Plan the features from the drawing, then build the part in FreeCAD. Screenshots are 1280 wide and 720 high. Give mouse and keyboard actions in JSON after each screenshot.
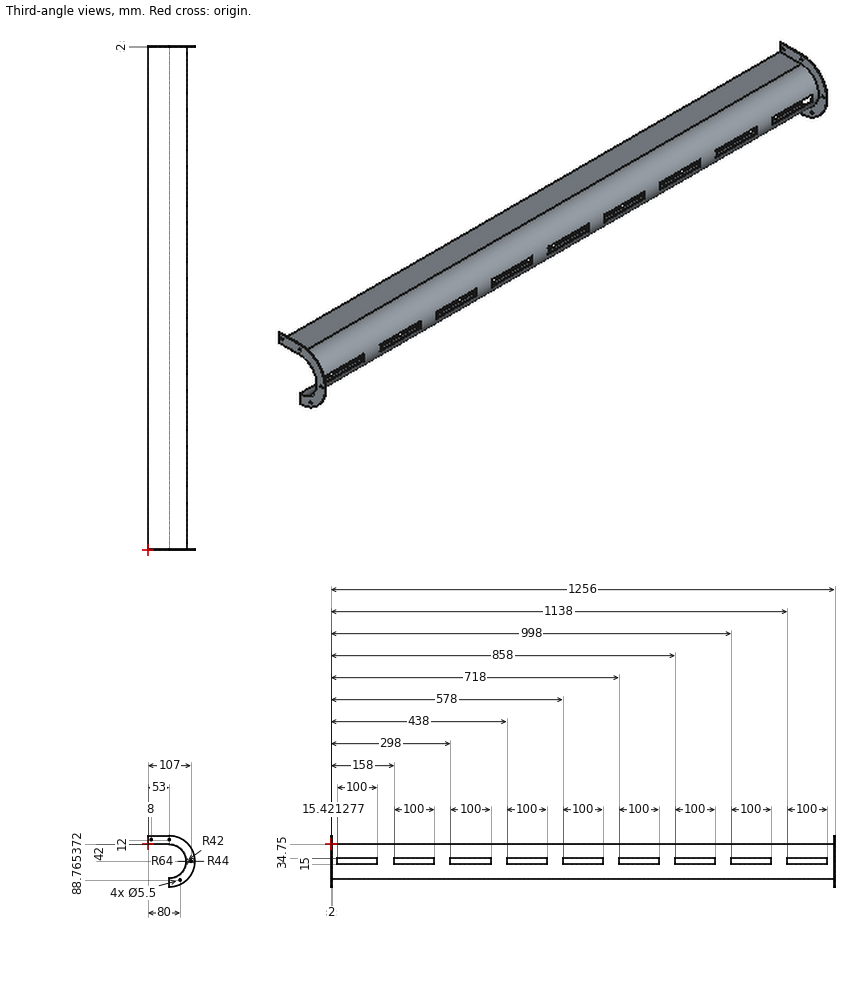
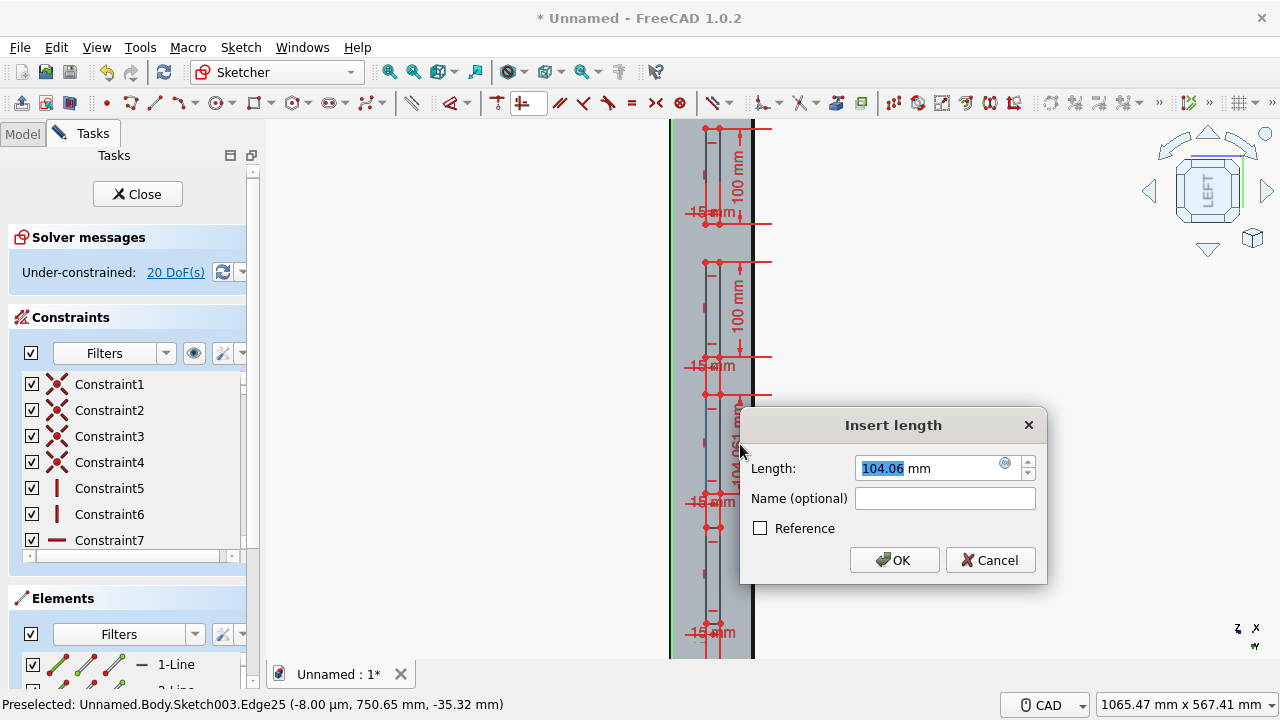
{"action": "type", "text": "100"}
{"action": "key", "text": "Return"}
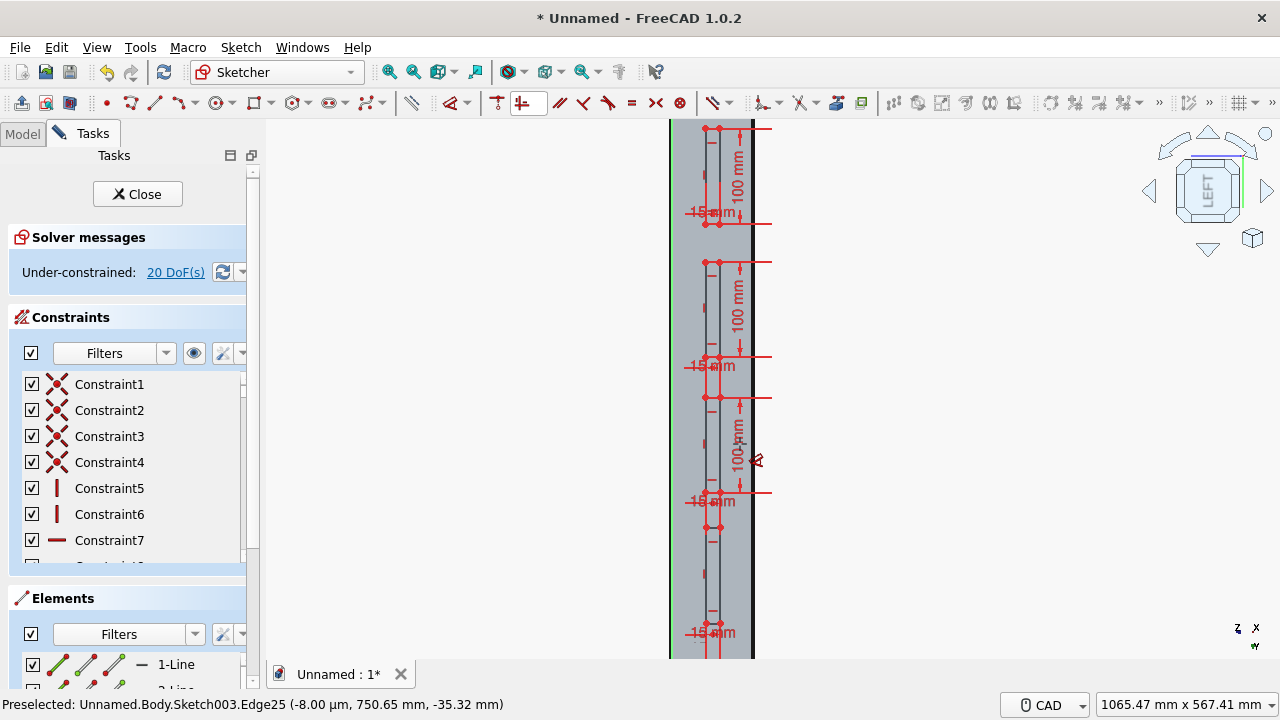
{"action": "left_click", "coordinate": [706, 557]}
{"action": "left_click", "coordinate": [740, 576]}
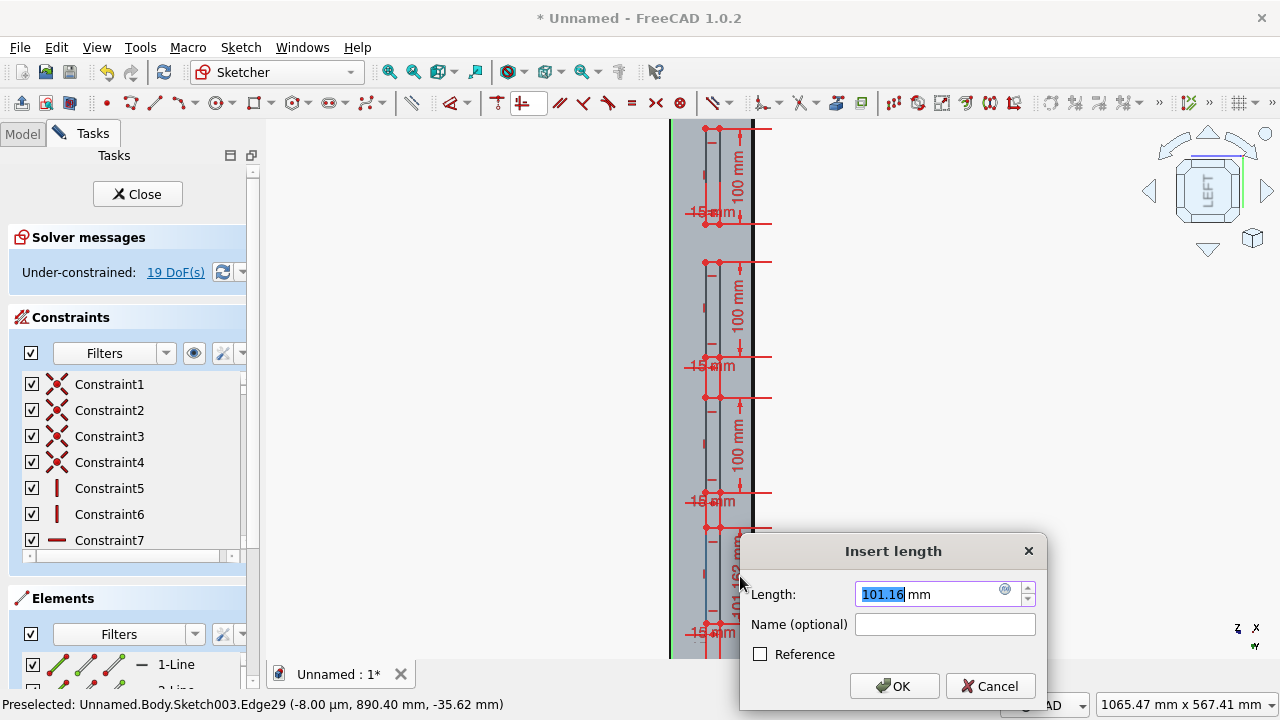
{"action": "type", "text": "100"}
{"action": "key", "text": "Return"}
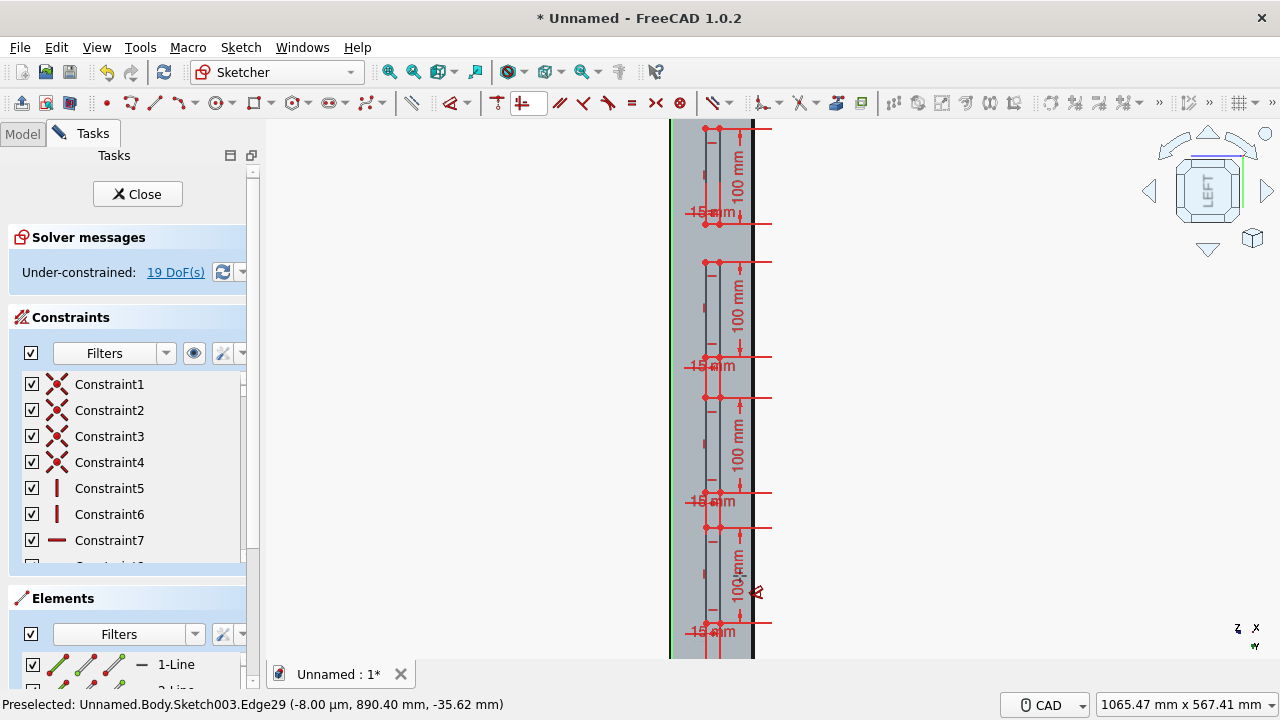
{"action": "scroll", "coordinate": [708, 427], "scroll_direction": "down", "scroll_amount": 6}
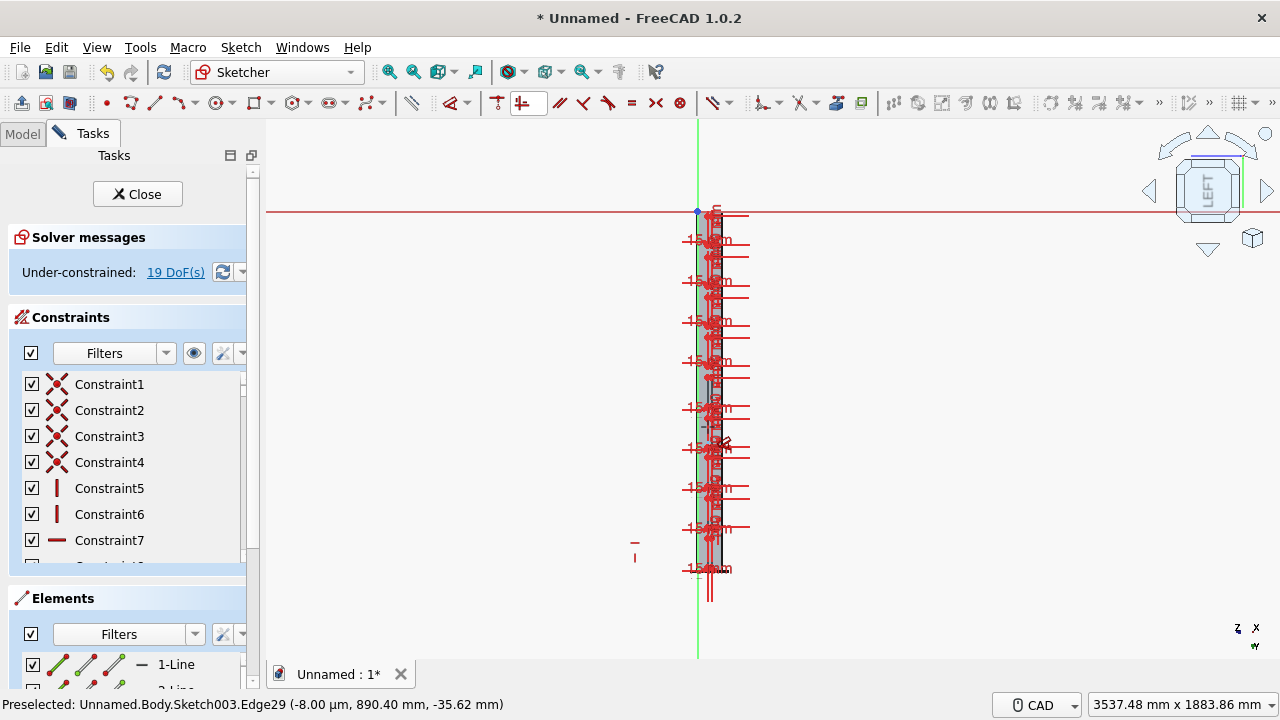
{"action": "scroll", "coordinate": [708, 547], "scroll_direction": "up", "scroll_amount": 6}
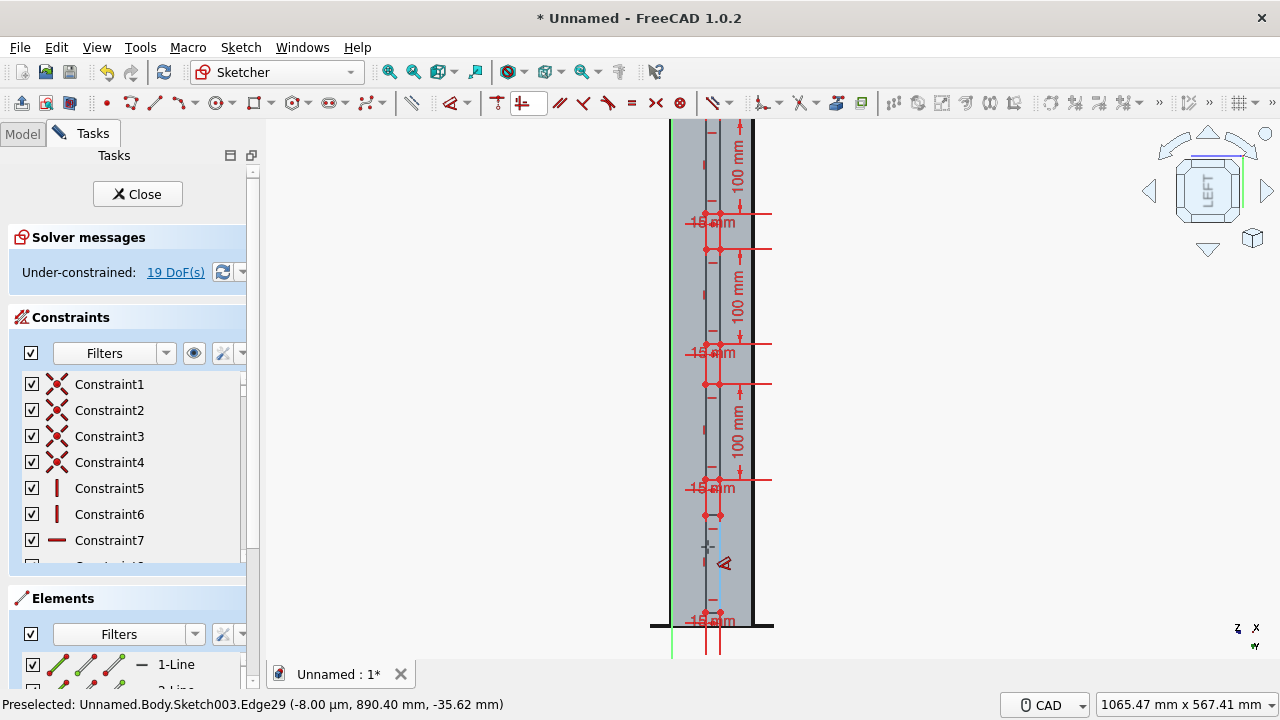
{"action": "left_click", "coordinate": [706, 544]}
{"action": "left_click", "coordinate": [740, 564]}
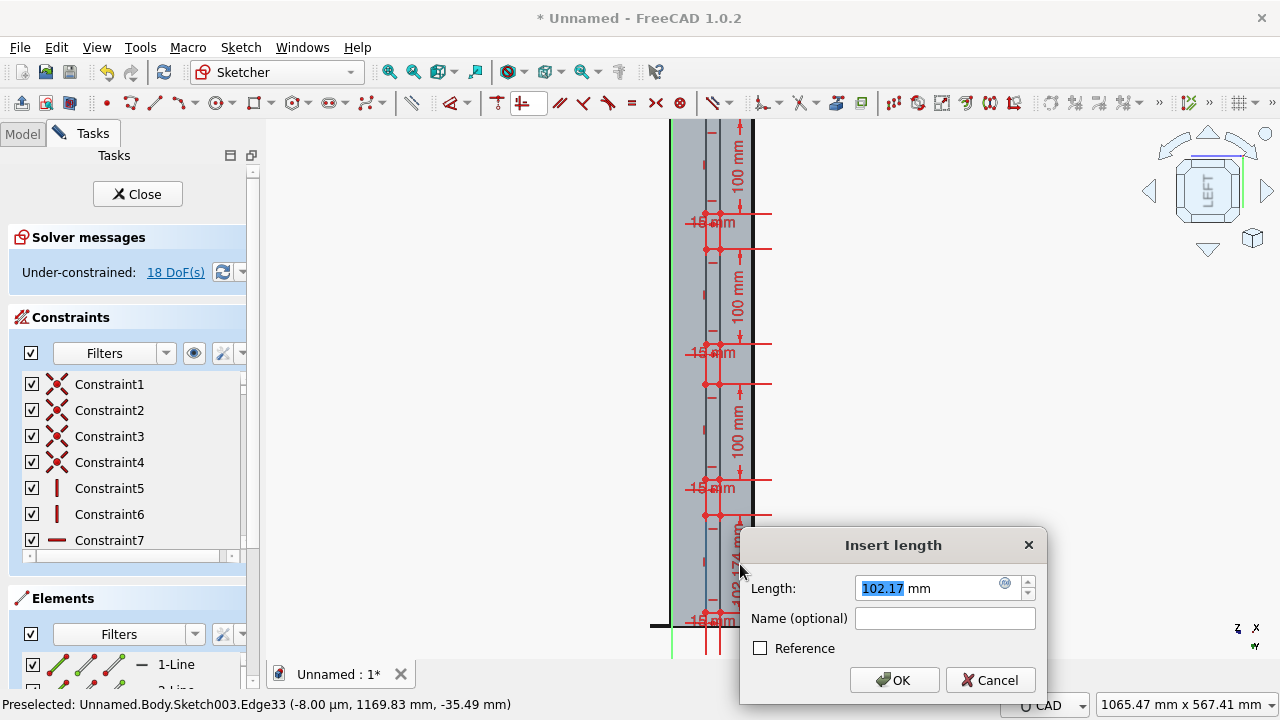
{"action": "type", "text": "100"}
{"action": "key", "text": "Return"}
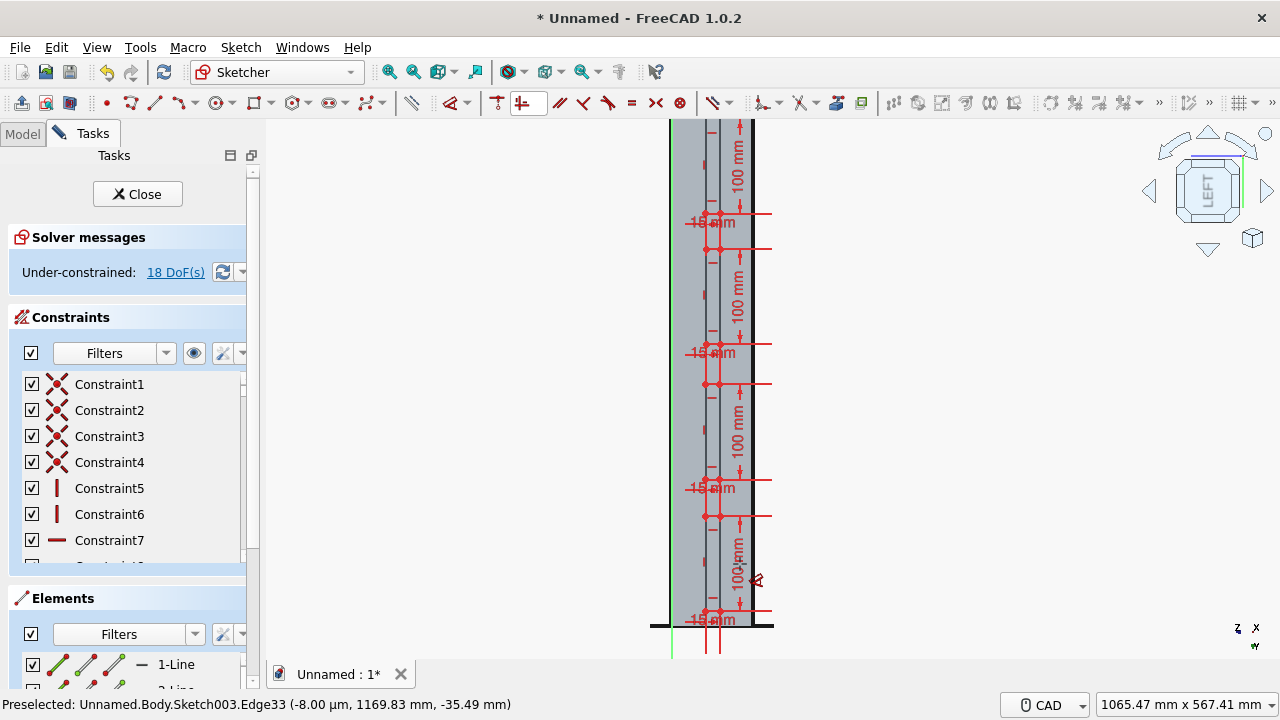
{"action": "scroll", "coordinate": [708, 548], "scroll_direction": "down", "scroll_amount": 6}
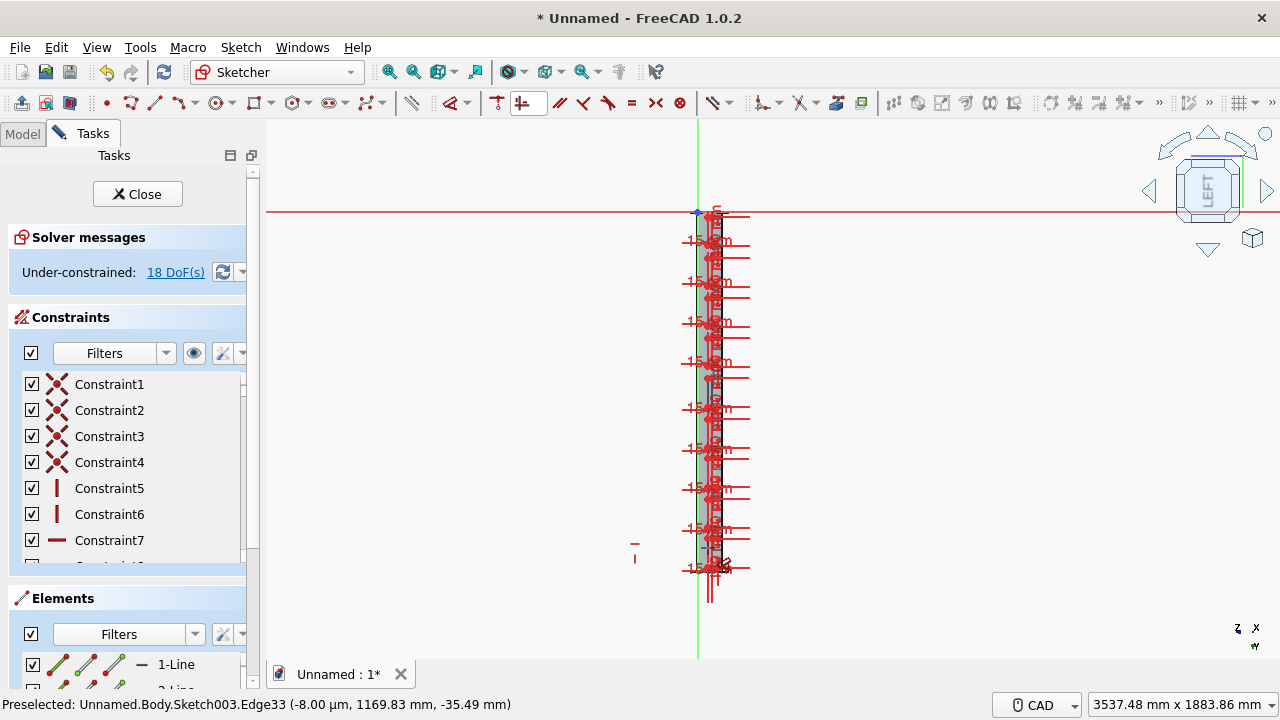
{"action": "scroll", "coordinate": [708, 258], "scroll_direction": "up", "scroll_amount": 6}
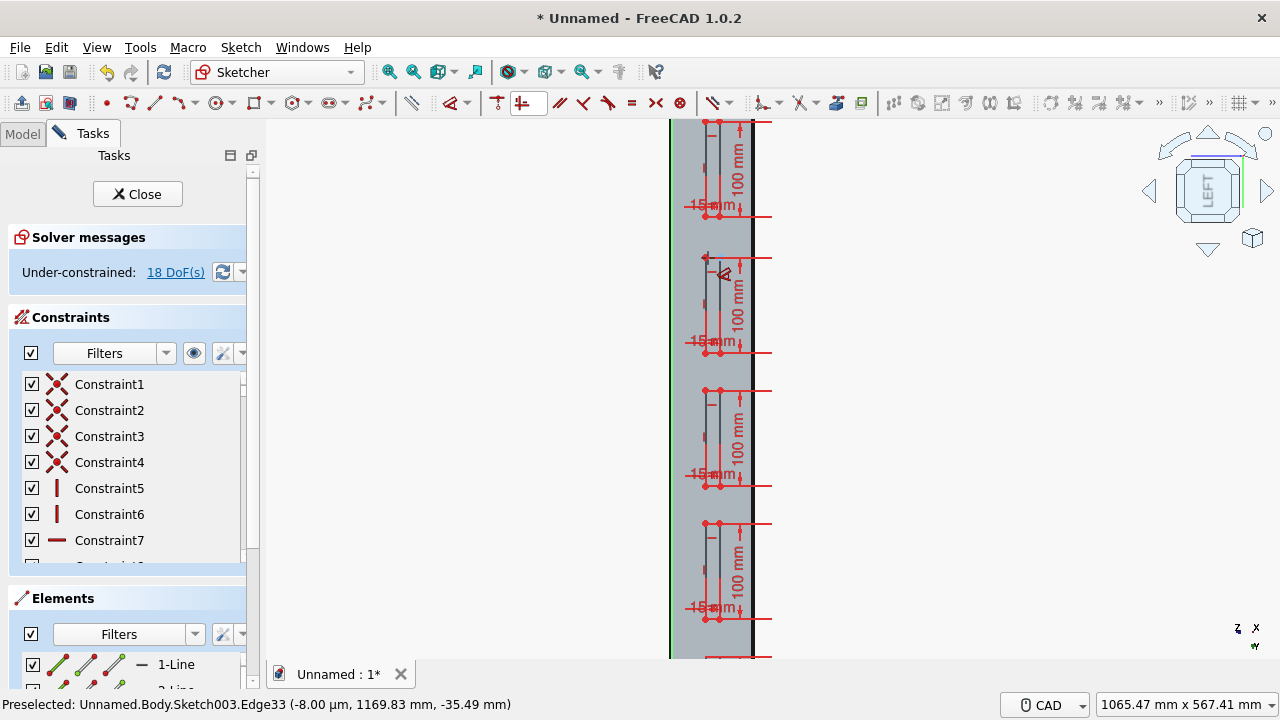
{"action": "left_click", "coordinate": [706, 258]}
{"action": "left_click", "coordinate": [638, 202]}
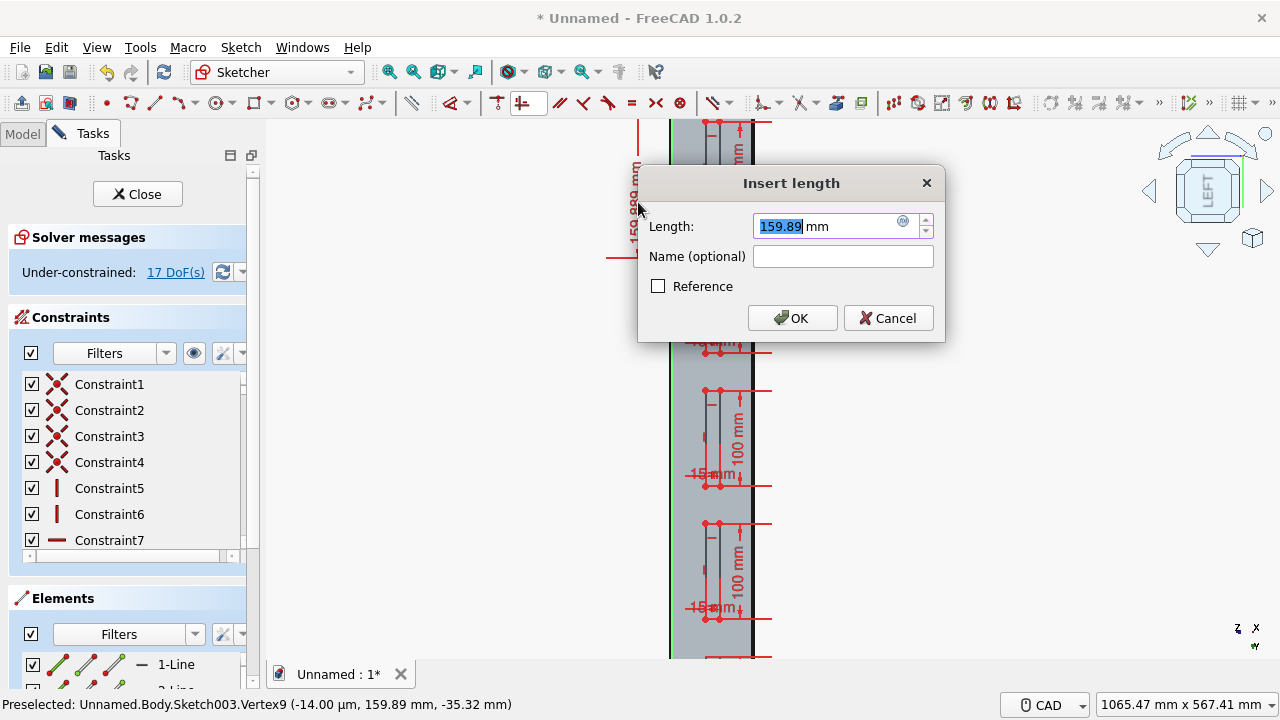
{"action": "type", "text": "158"}
{"action": "key", "text": "Return"}